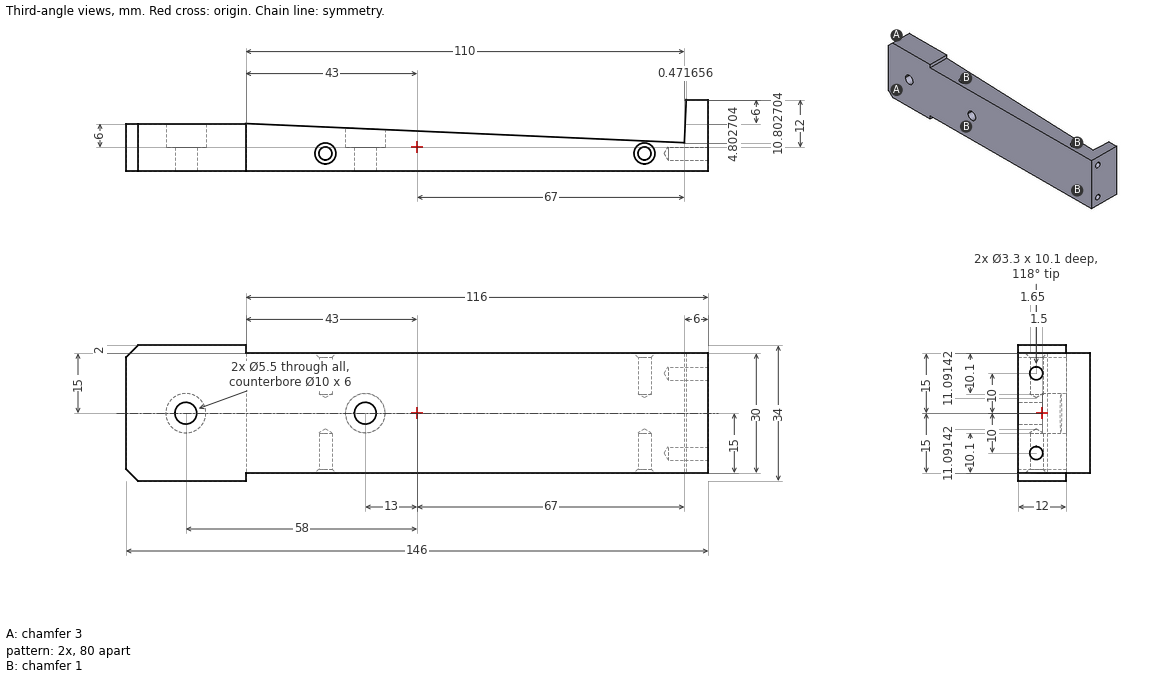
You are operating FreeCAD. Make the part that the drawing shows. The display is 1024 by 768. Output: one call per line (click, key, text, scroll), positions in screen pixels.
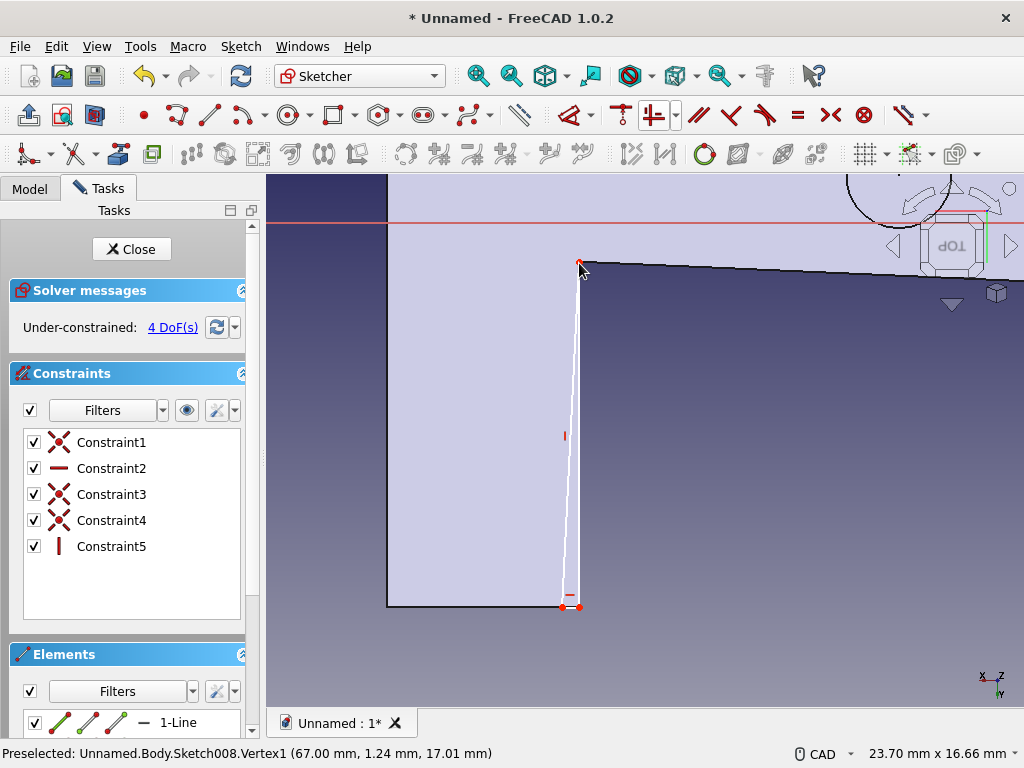
key(d)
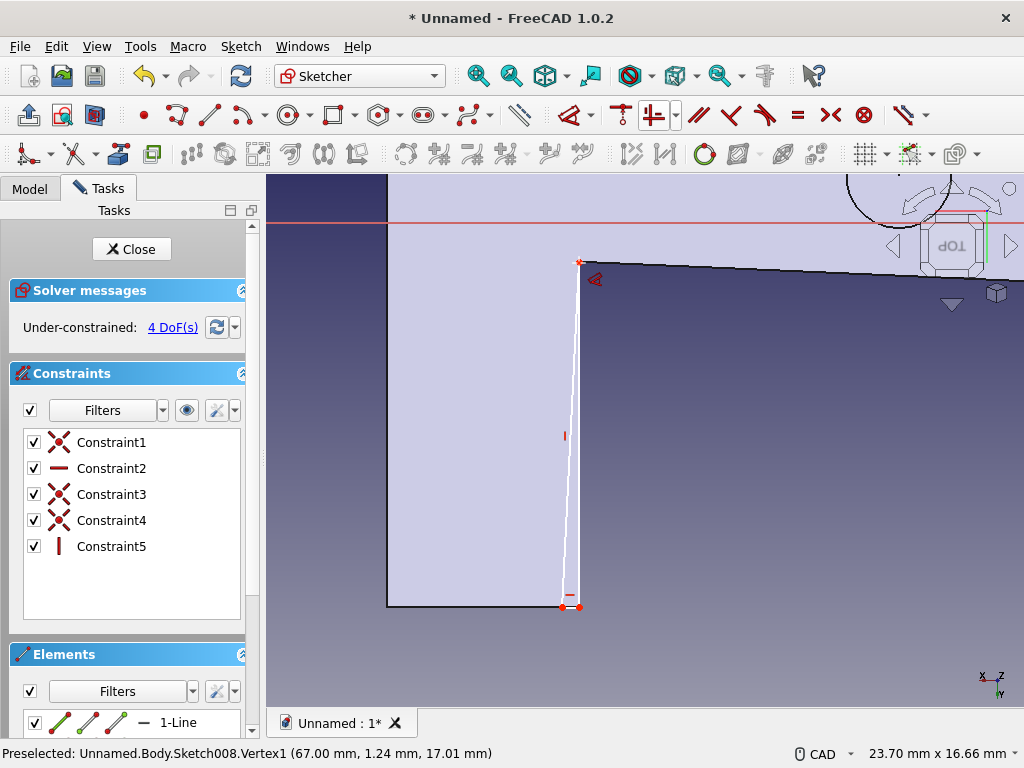
click(579, 263)
click(719, 297)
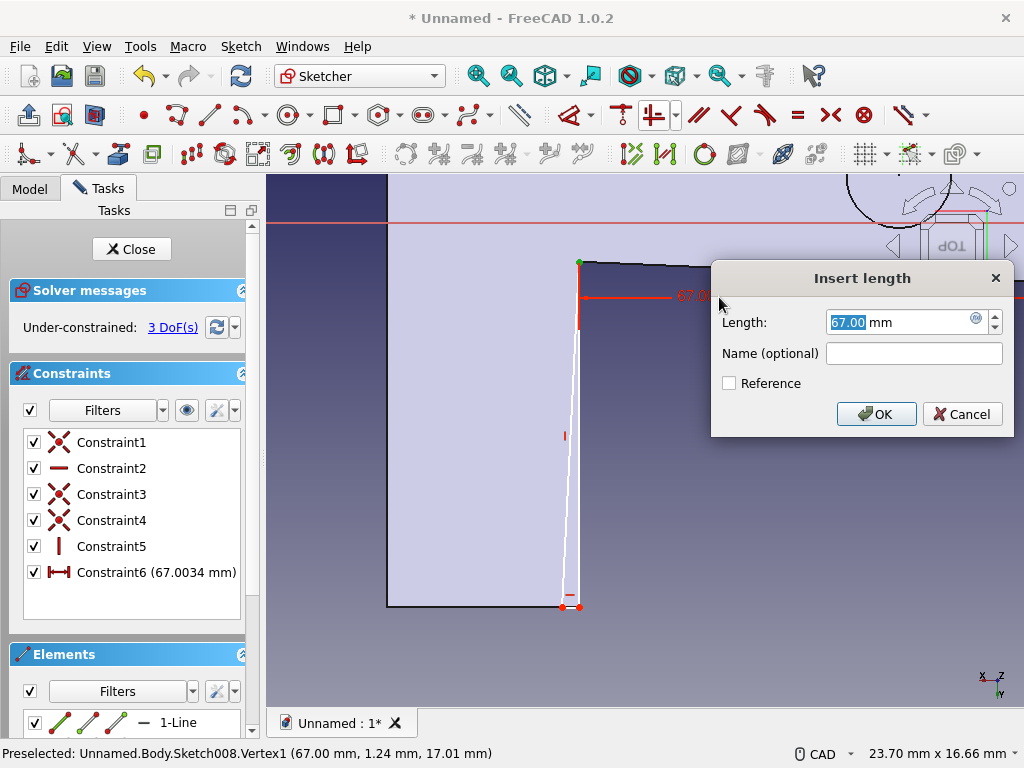
text(67)
key(Return)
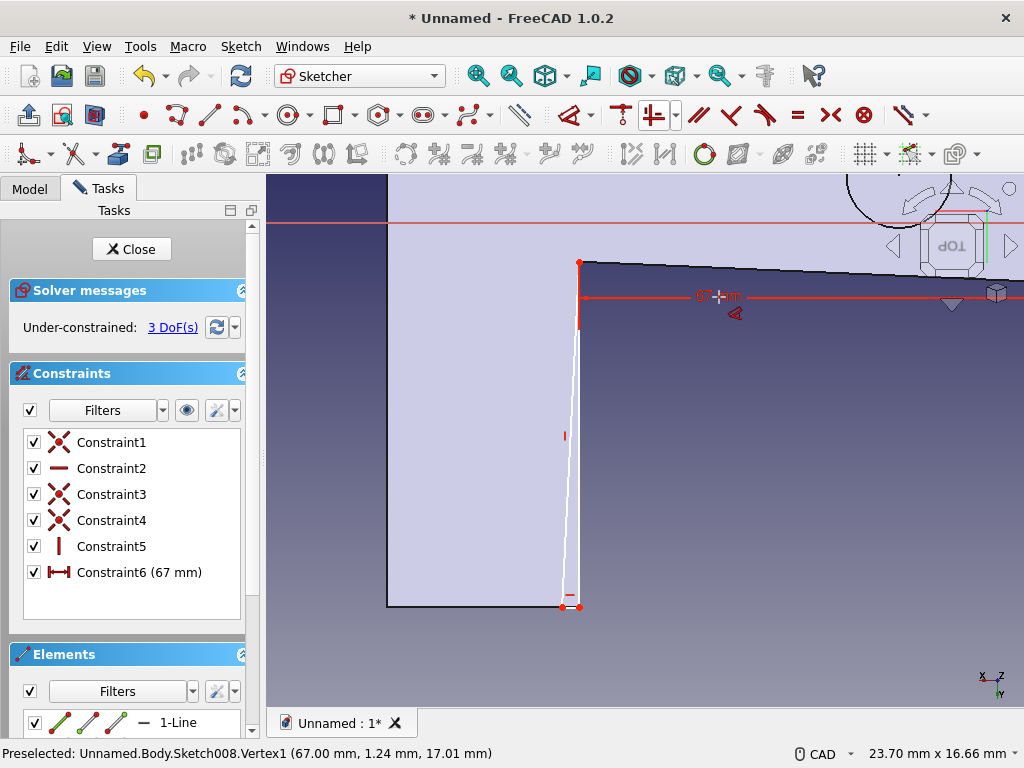
click(562, 608)
click(528, 416)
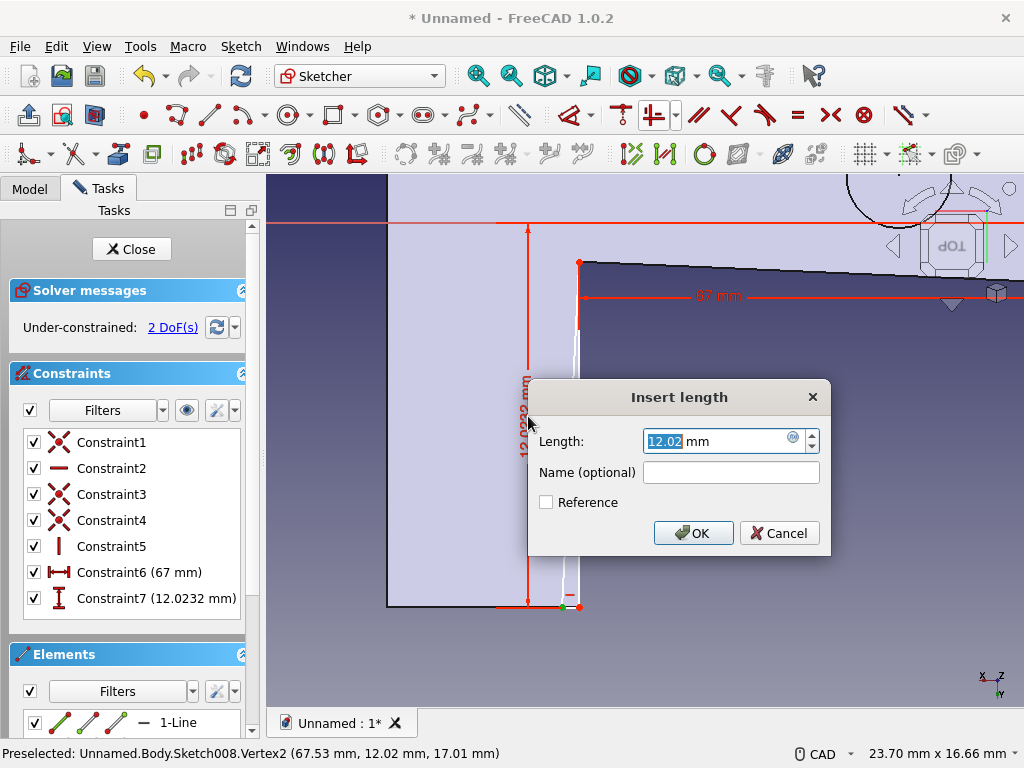
text(12)
key(Return)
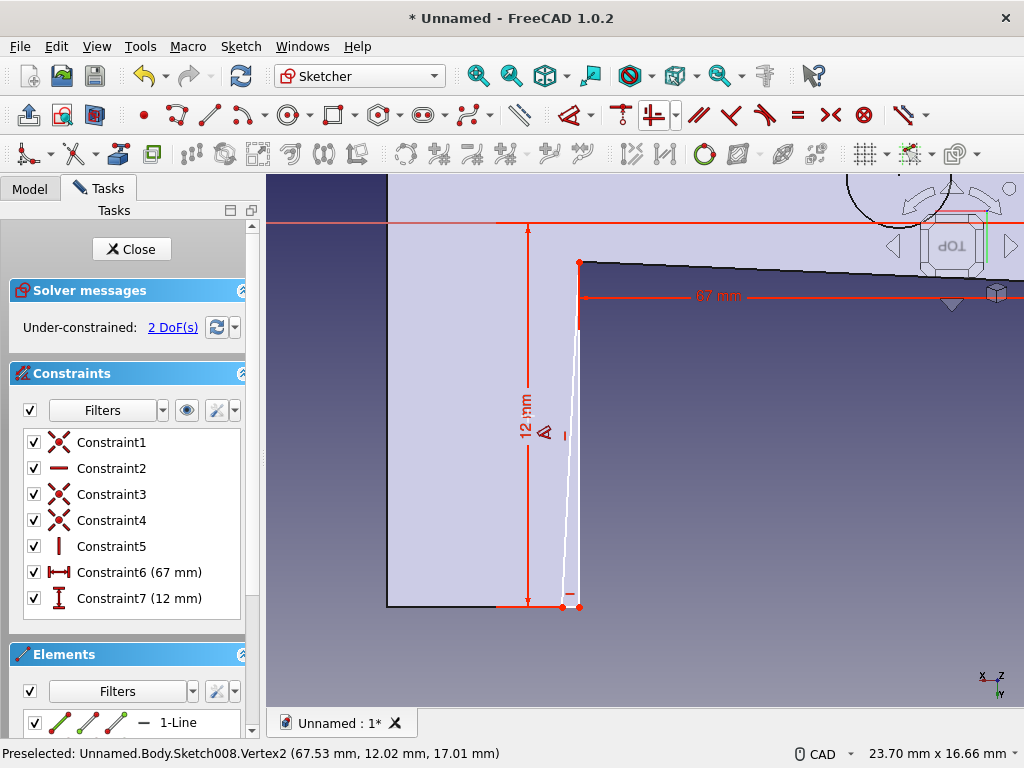
scroll(571, 607, up, 5)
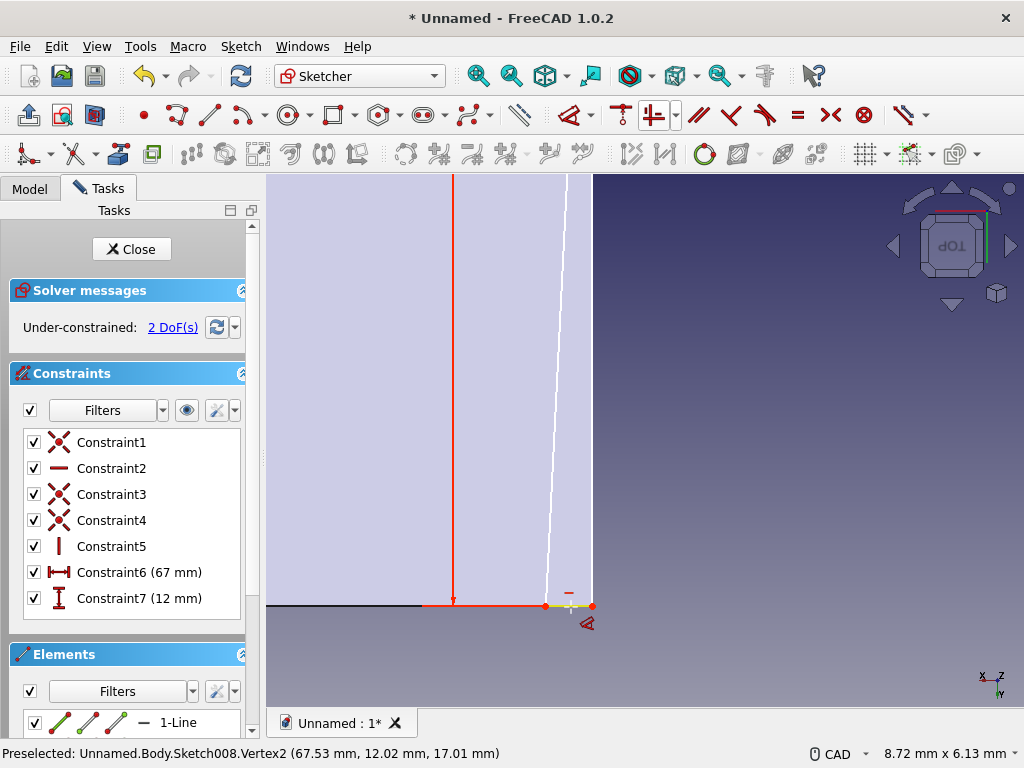
click(569, 606)
click(569, 640)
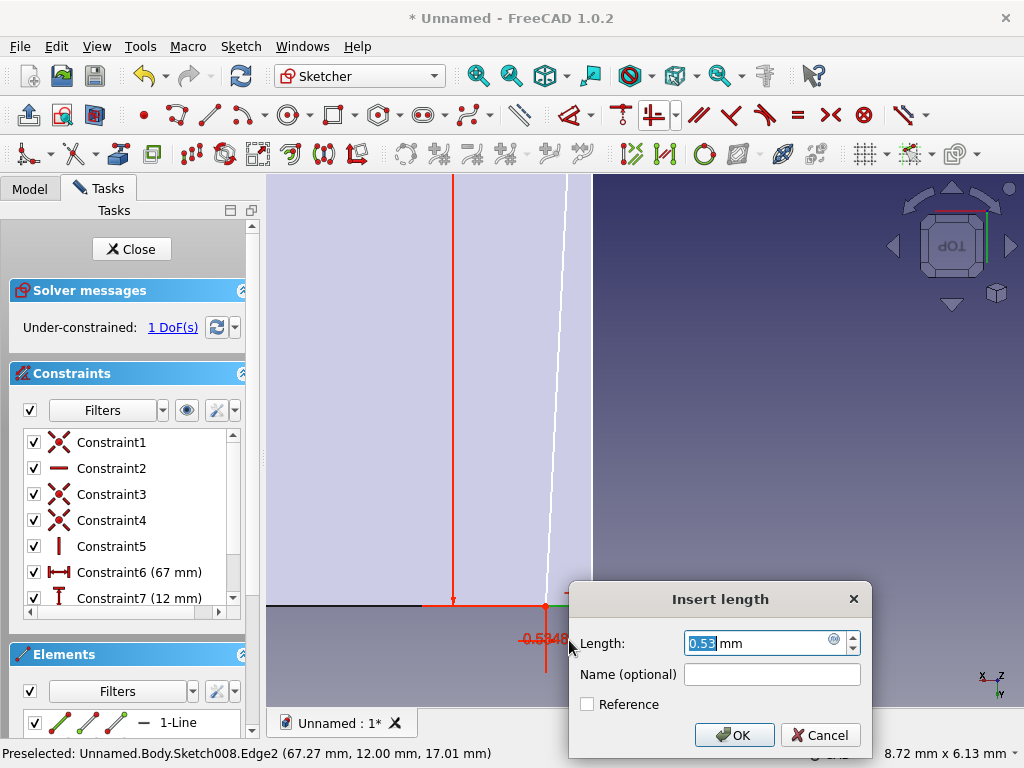
text(0.471656)
key(Return)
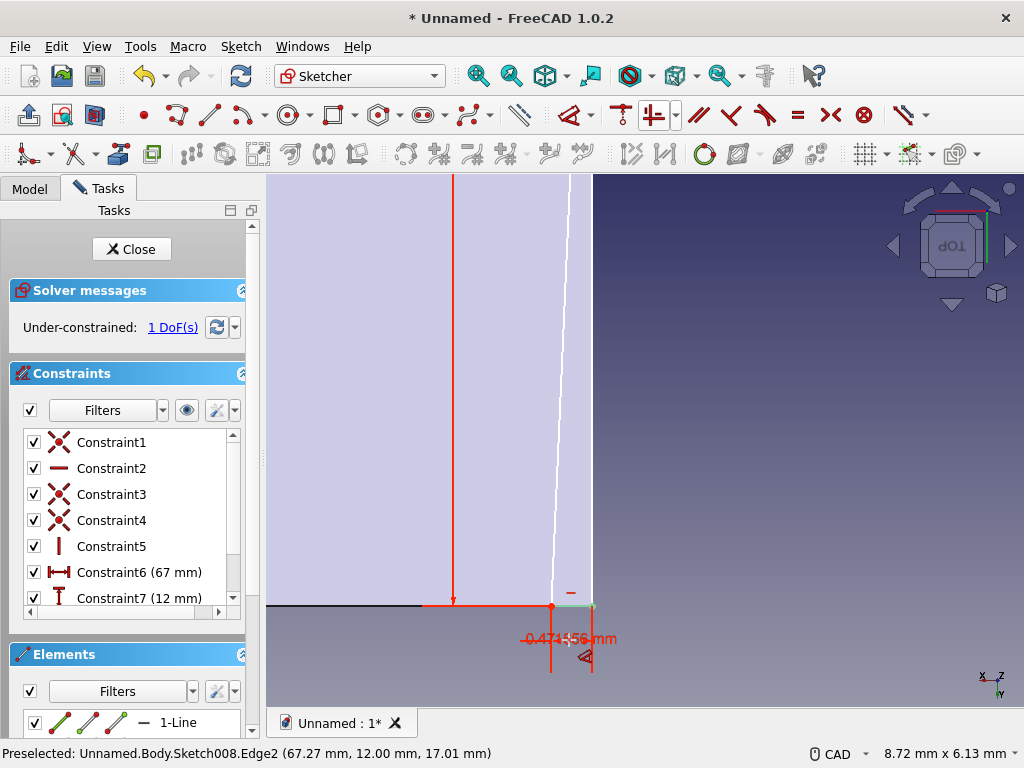
click(592, 326)
click(626, 404)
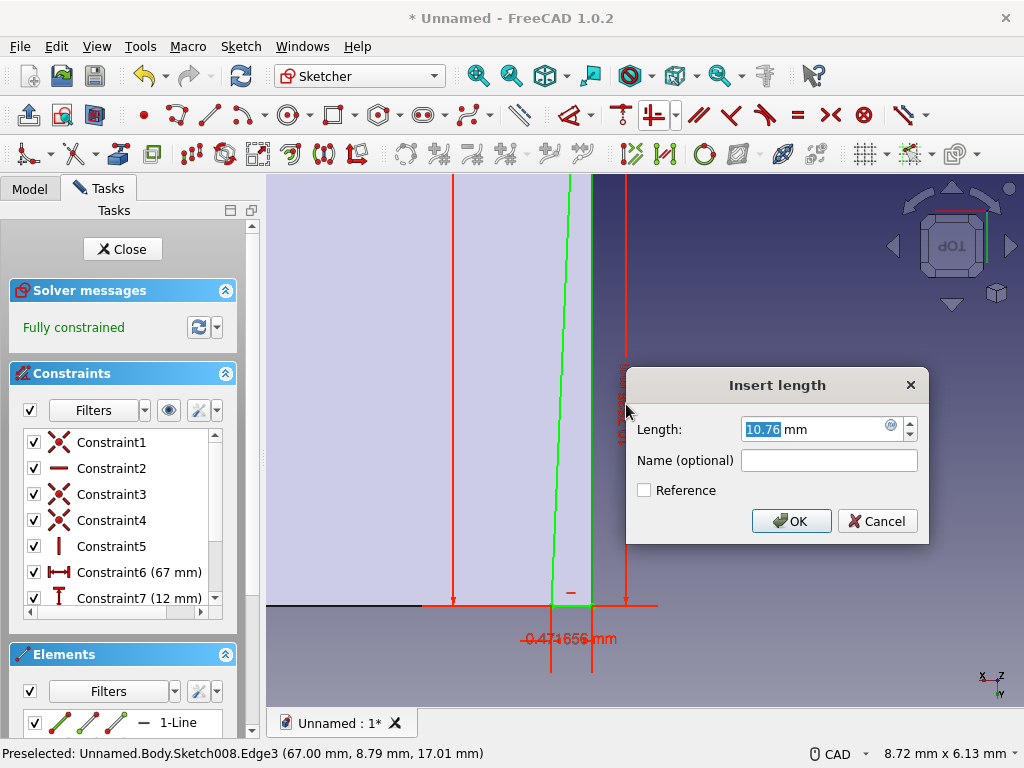
text(10.802704)
key(Return)
key(Escape)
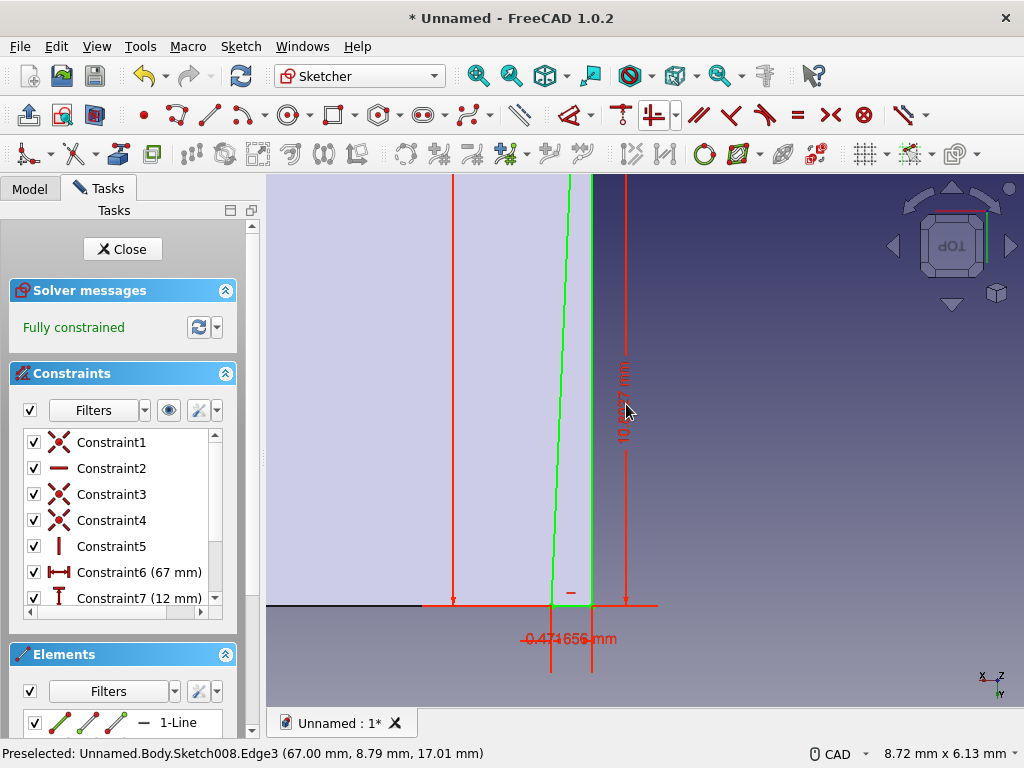
click(123, 249)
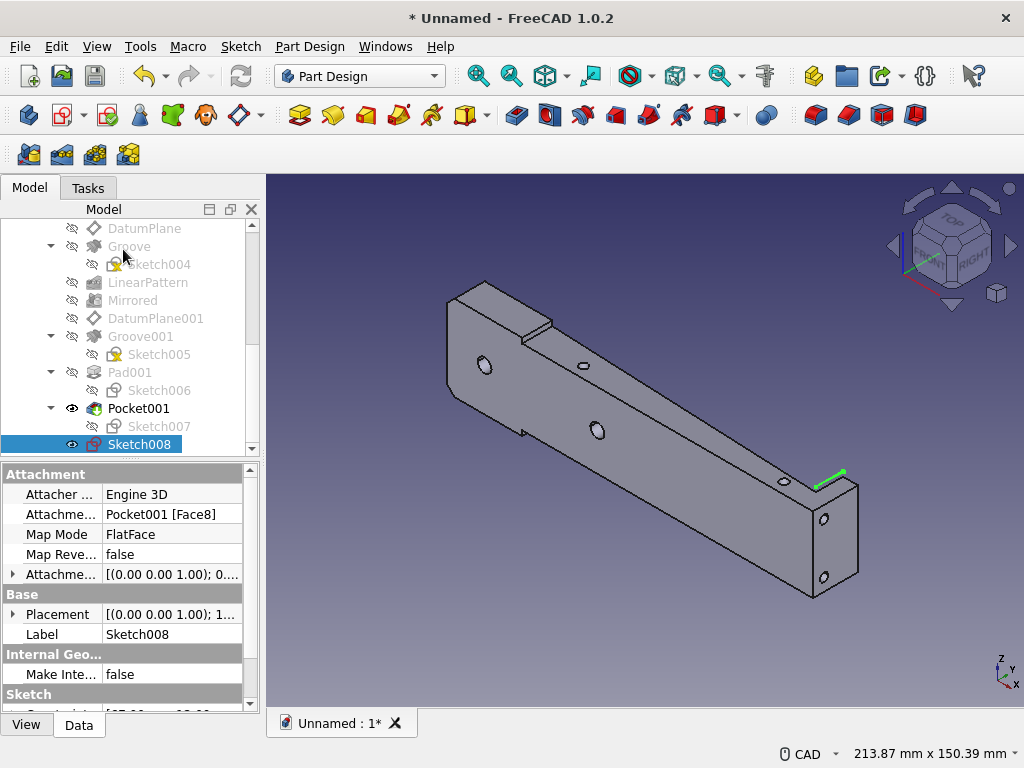
click(517, 116)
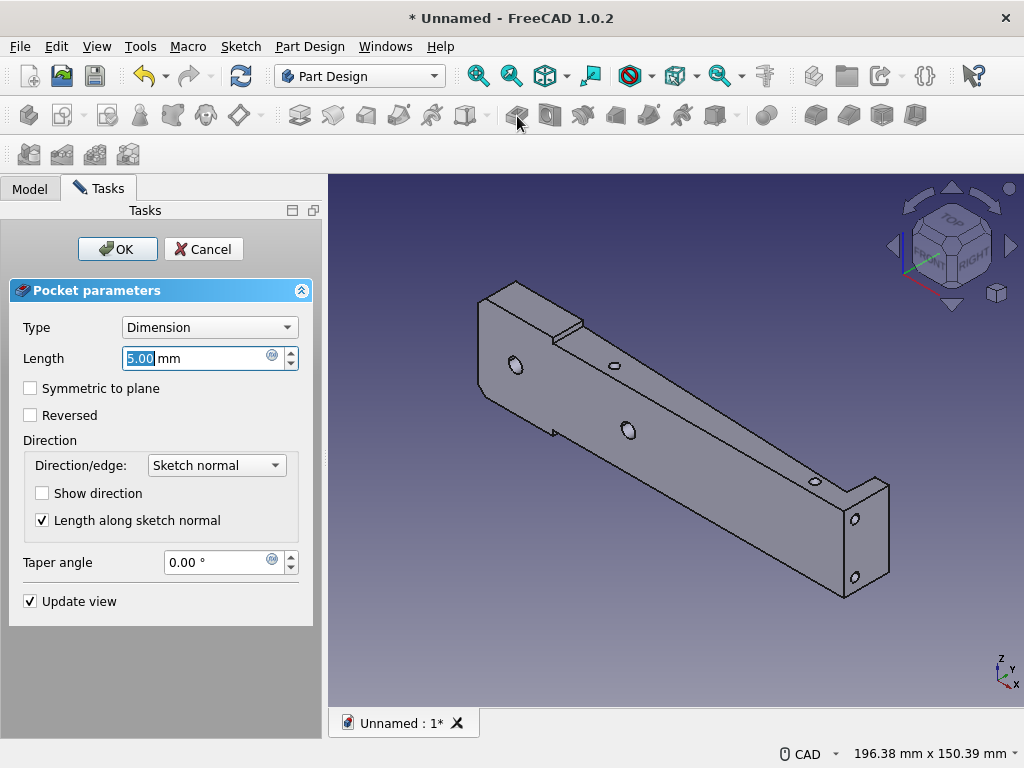
click(210, 328)